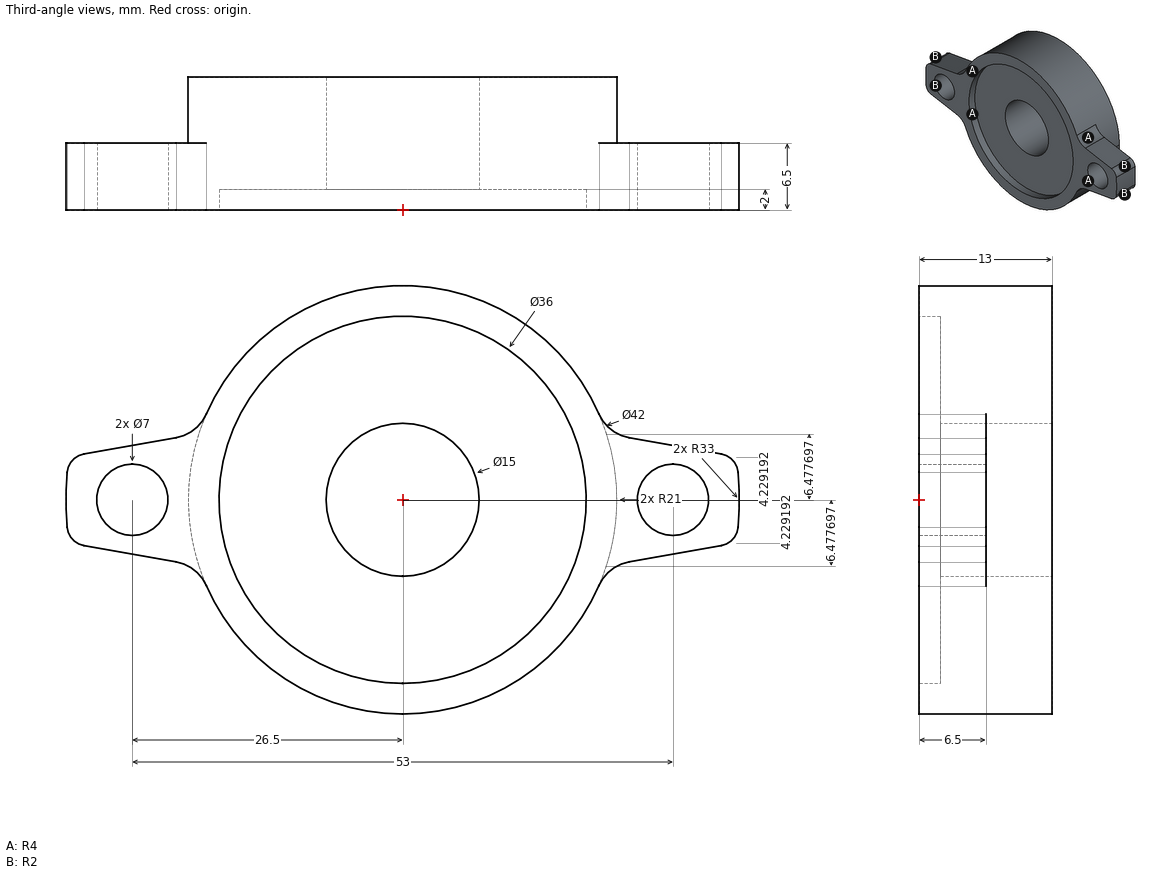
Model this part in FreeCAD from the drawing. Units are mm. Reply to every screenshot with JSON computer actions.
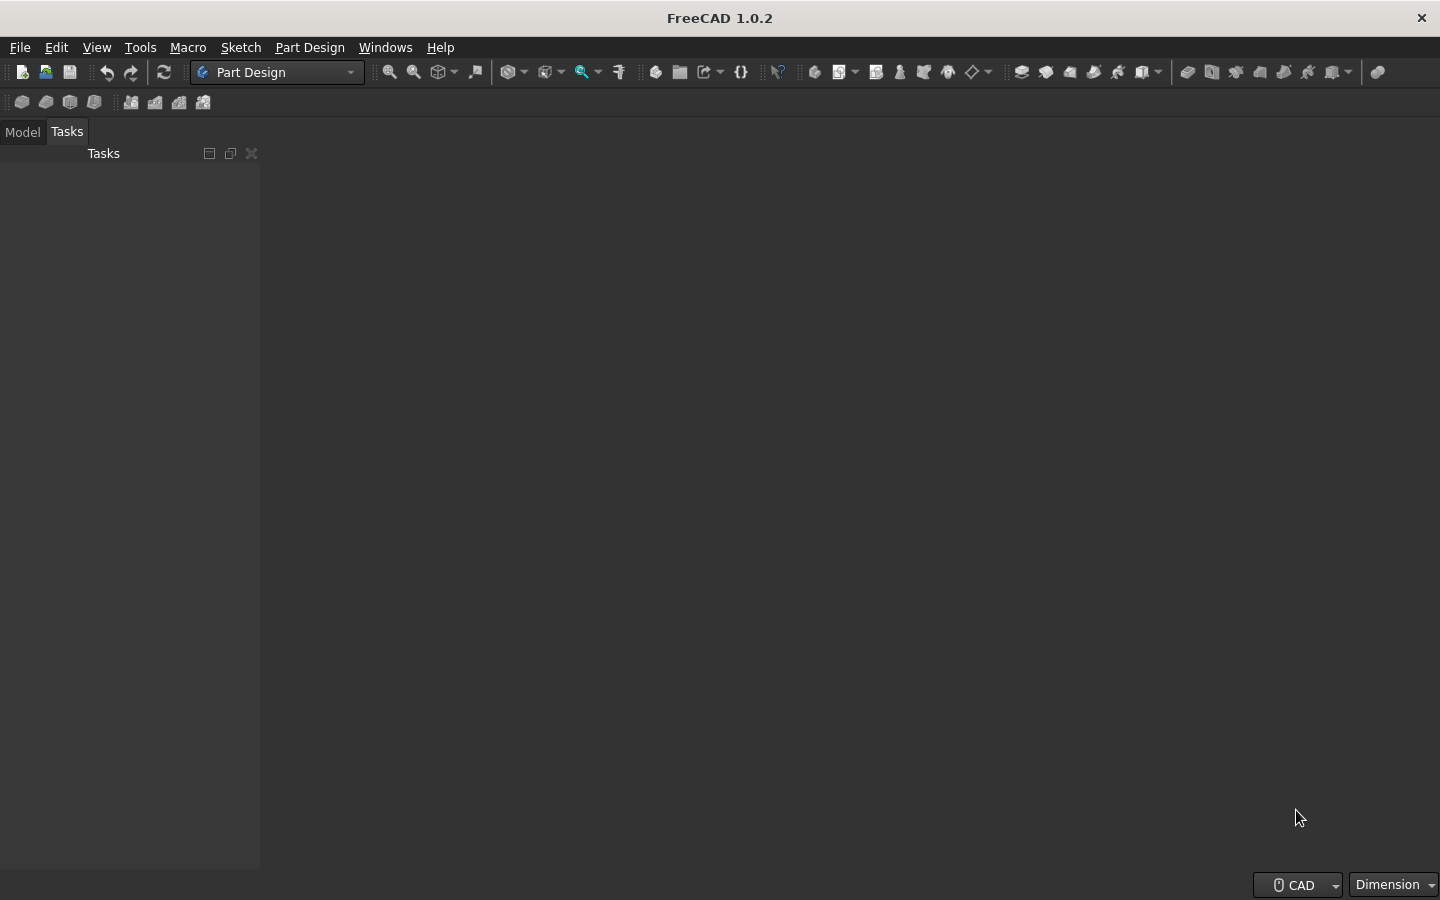
{"action": "left_click", "coordinate": [22, 72]}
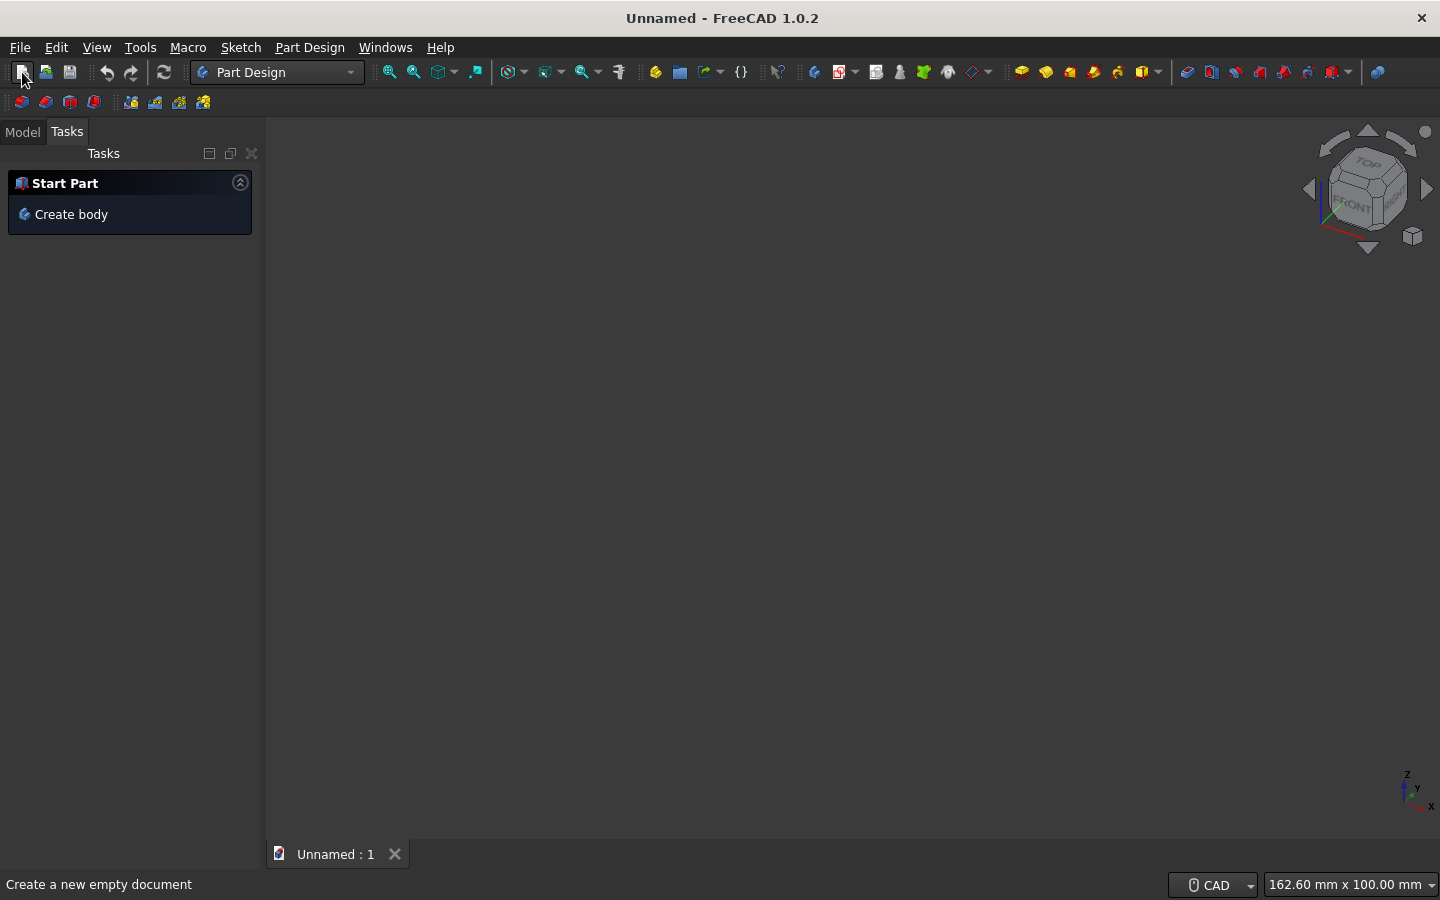
{"action": "left_click", "coordinate": [840, 72]}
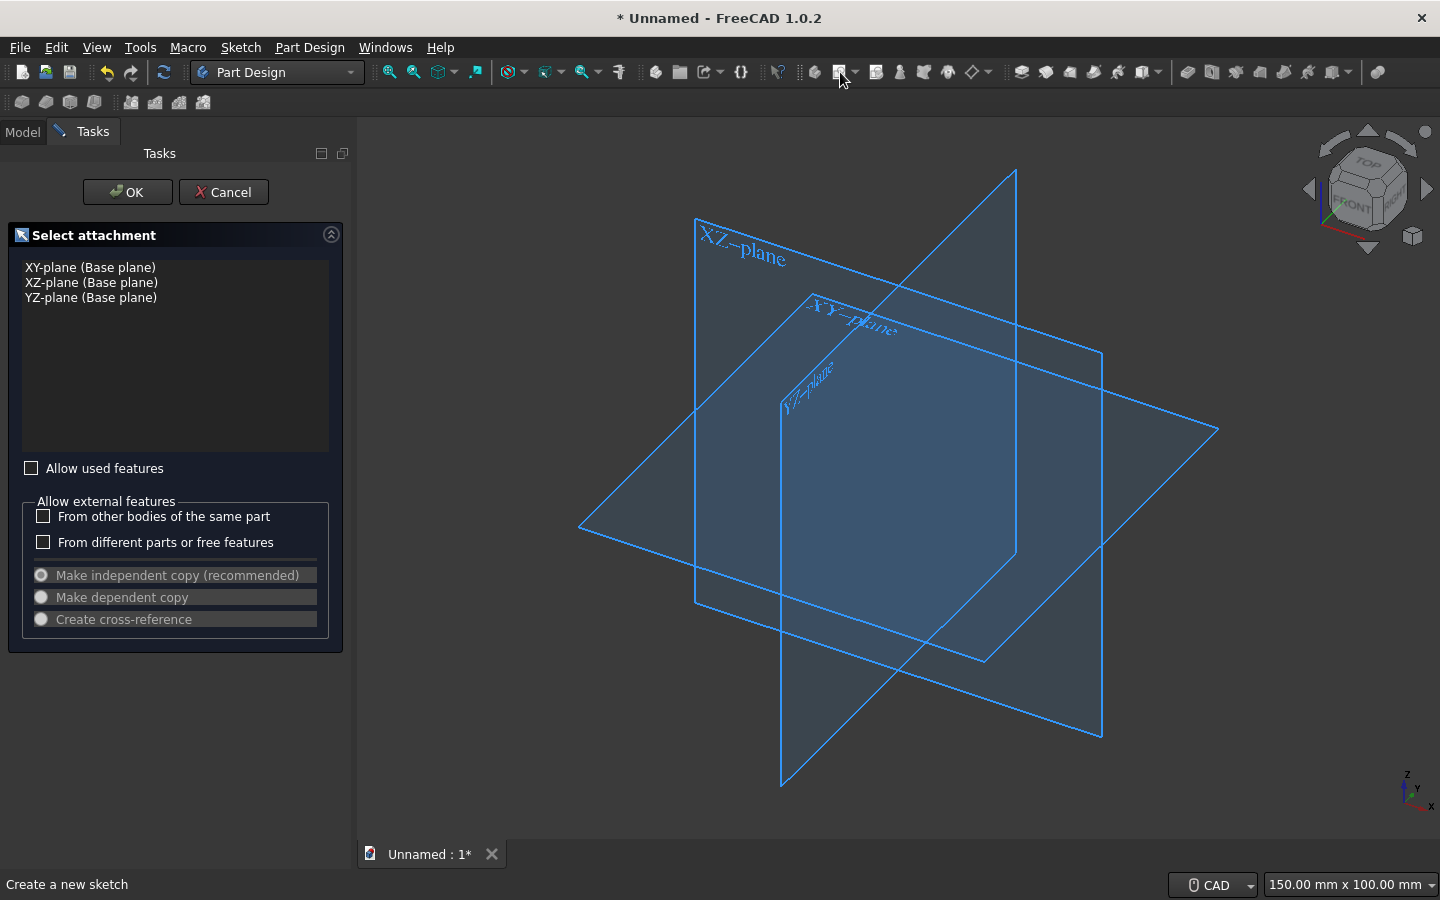
{"action": "left_click", "coordinate": [82, 282]}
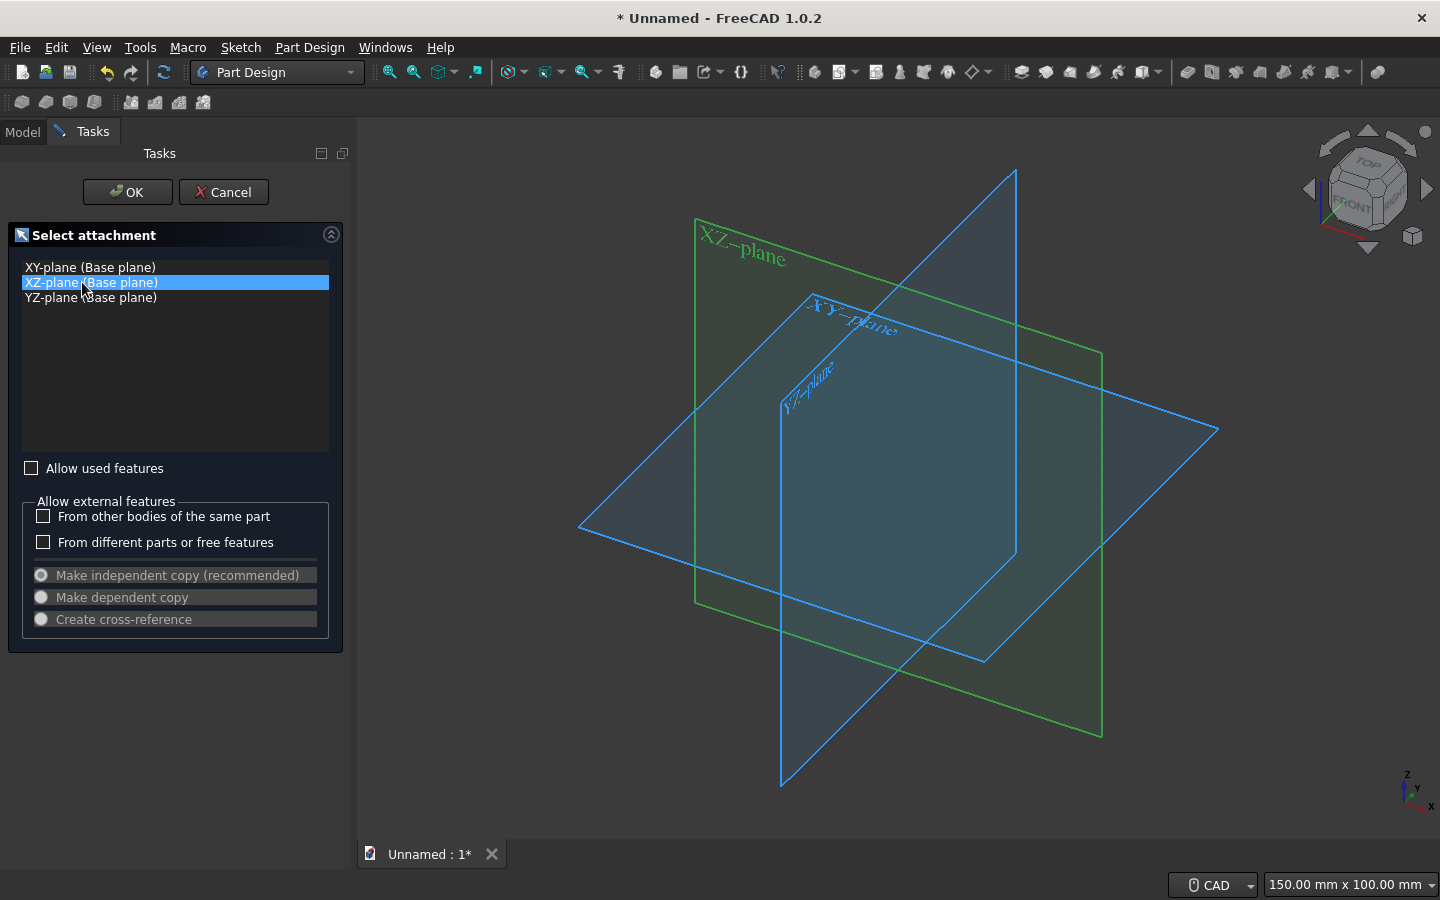
{"action": "left_click", "coordinate": [128, 192]}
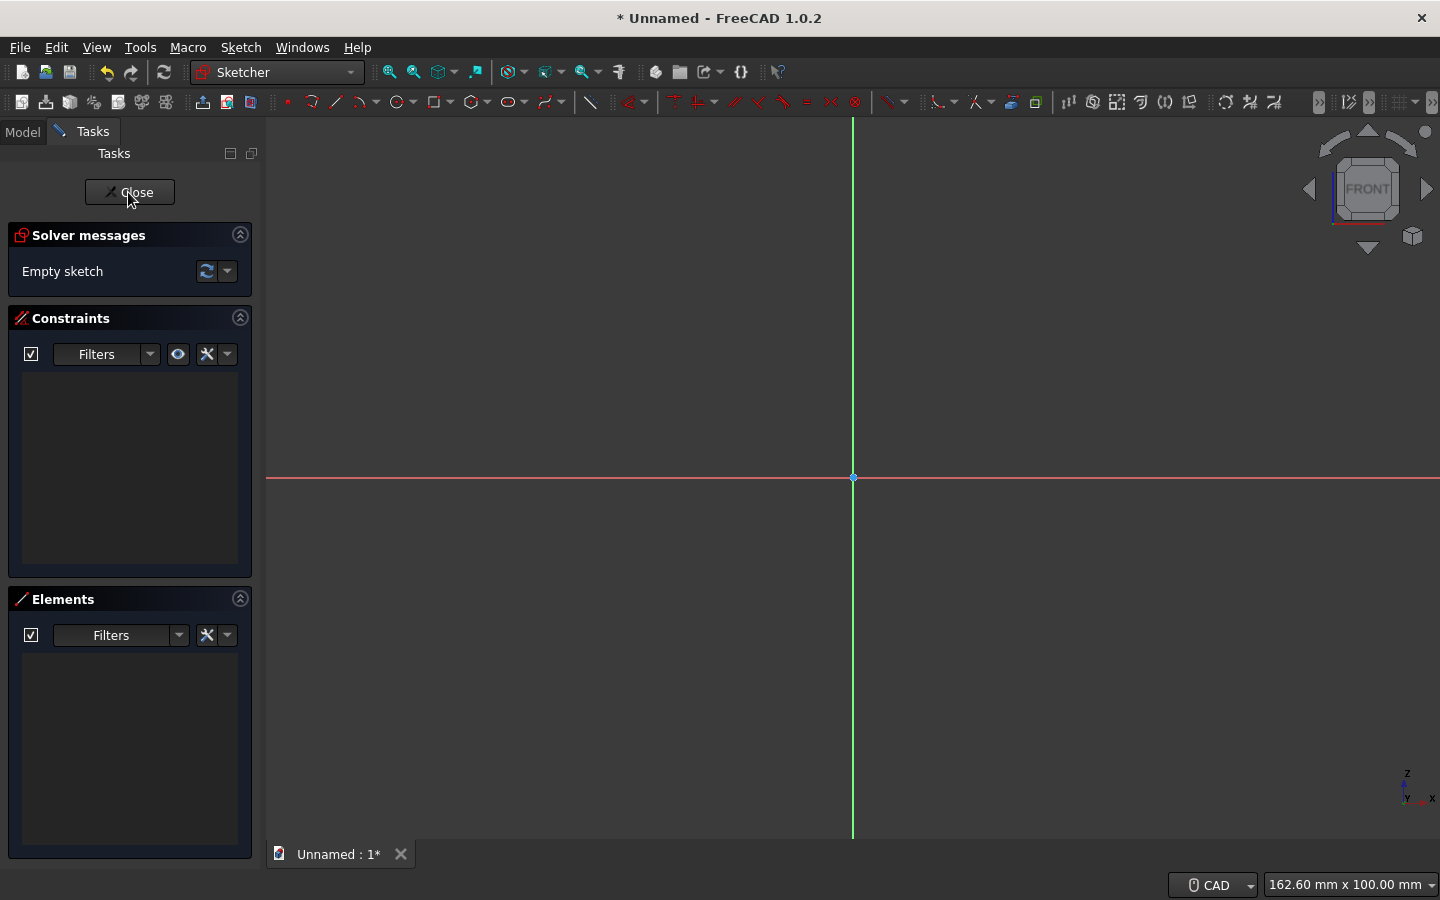
{"action": "scroll", "coordinate": [992, 478], "scroll_direction": "up", "scroll_amount": 2}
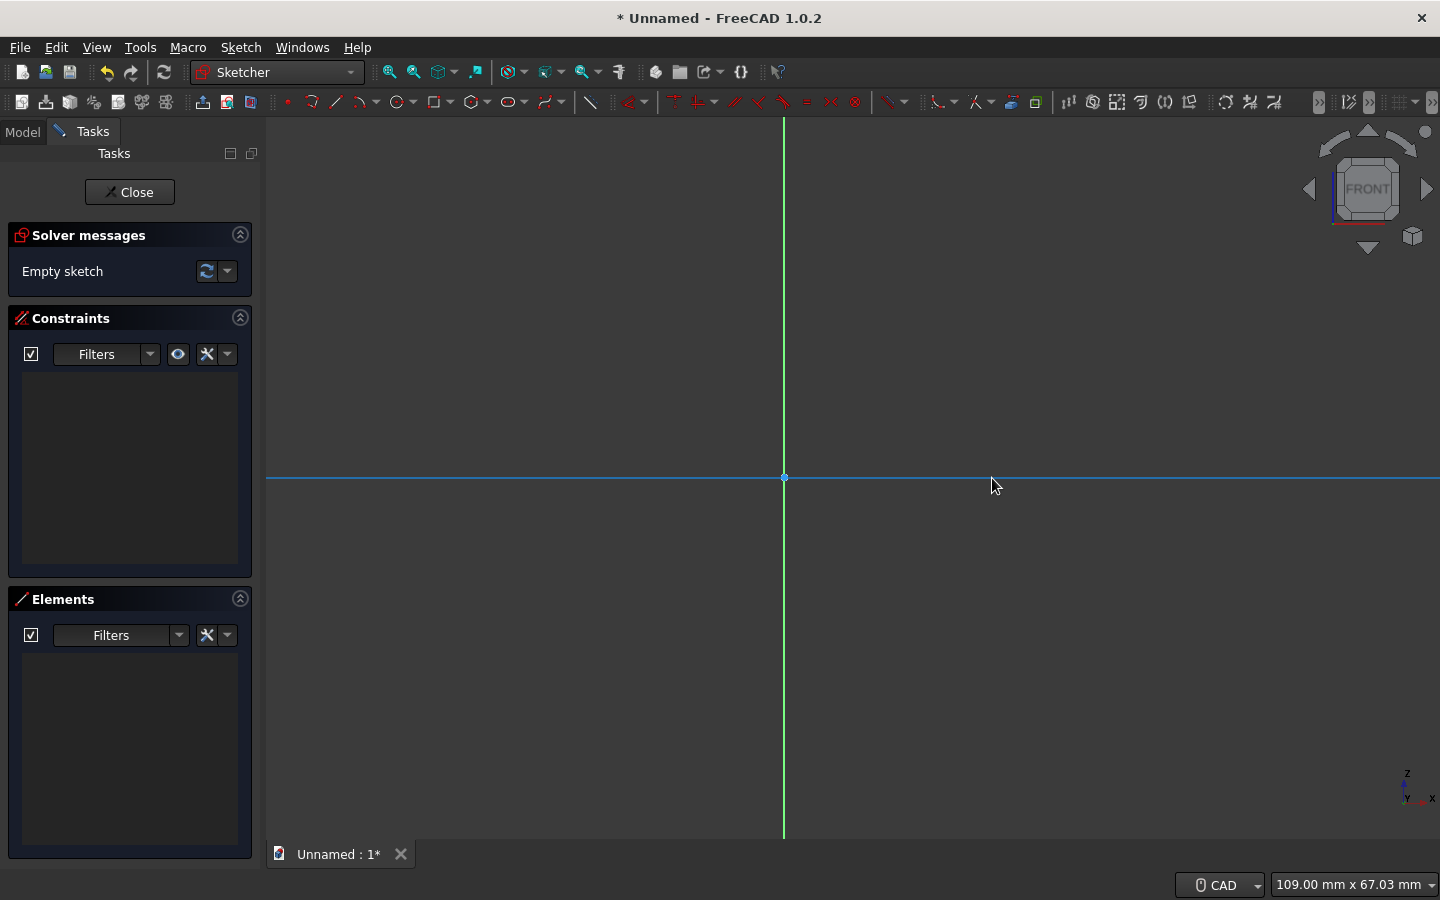
{"action": "left_click", "coordinate": [398, 102]}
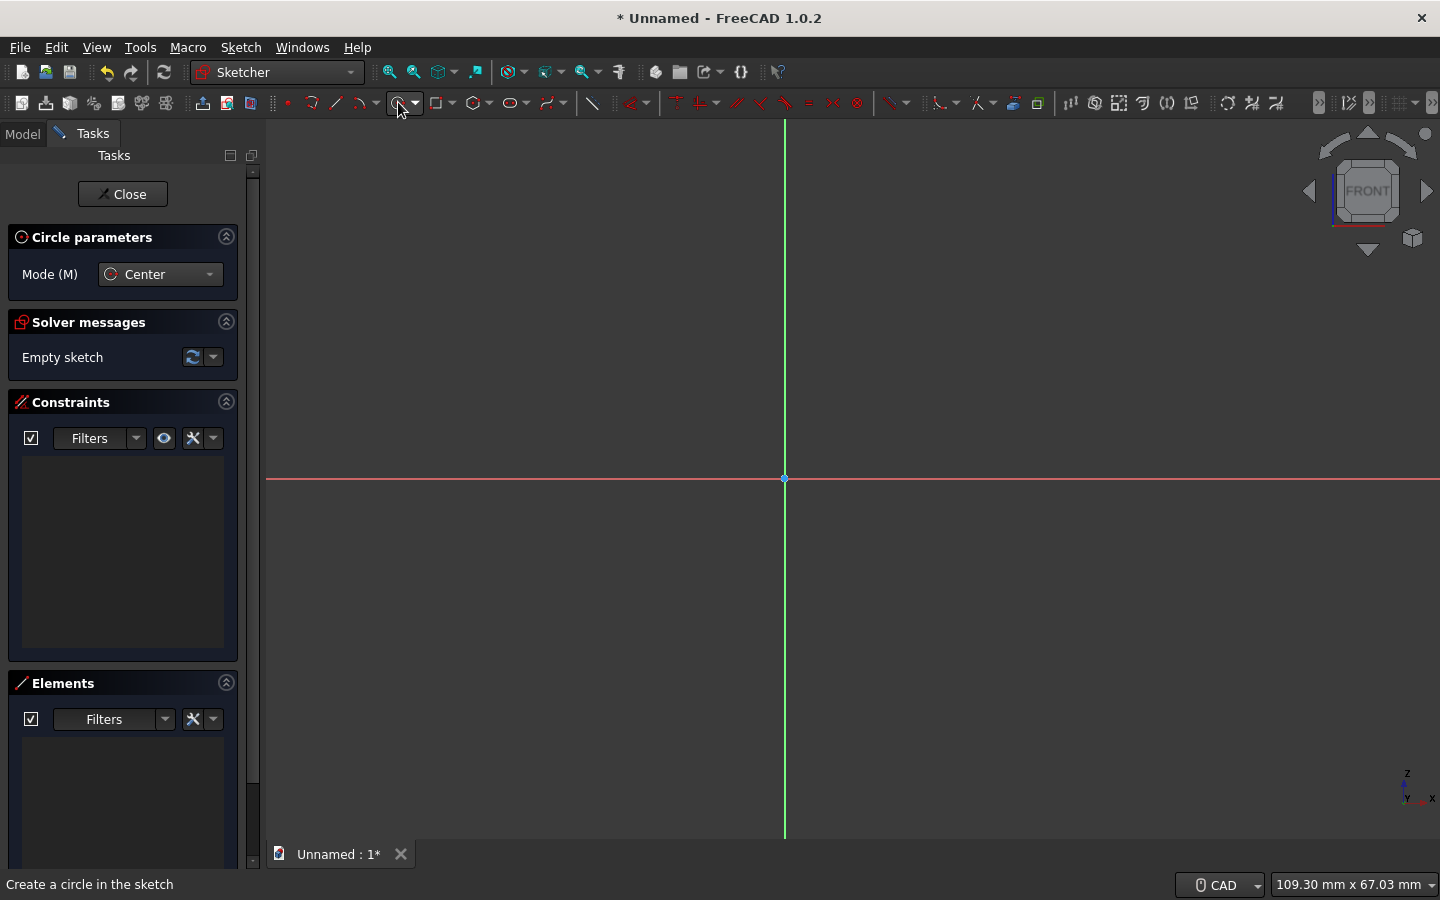
{"action": "left_click", "coordinate": [785, 479]}
{"action": "mouse_move", "coordinate": [944, 319]}